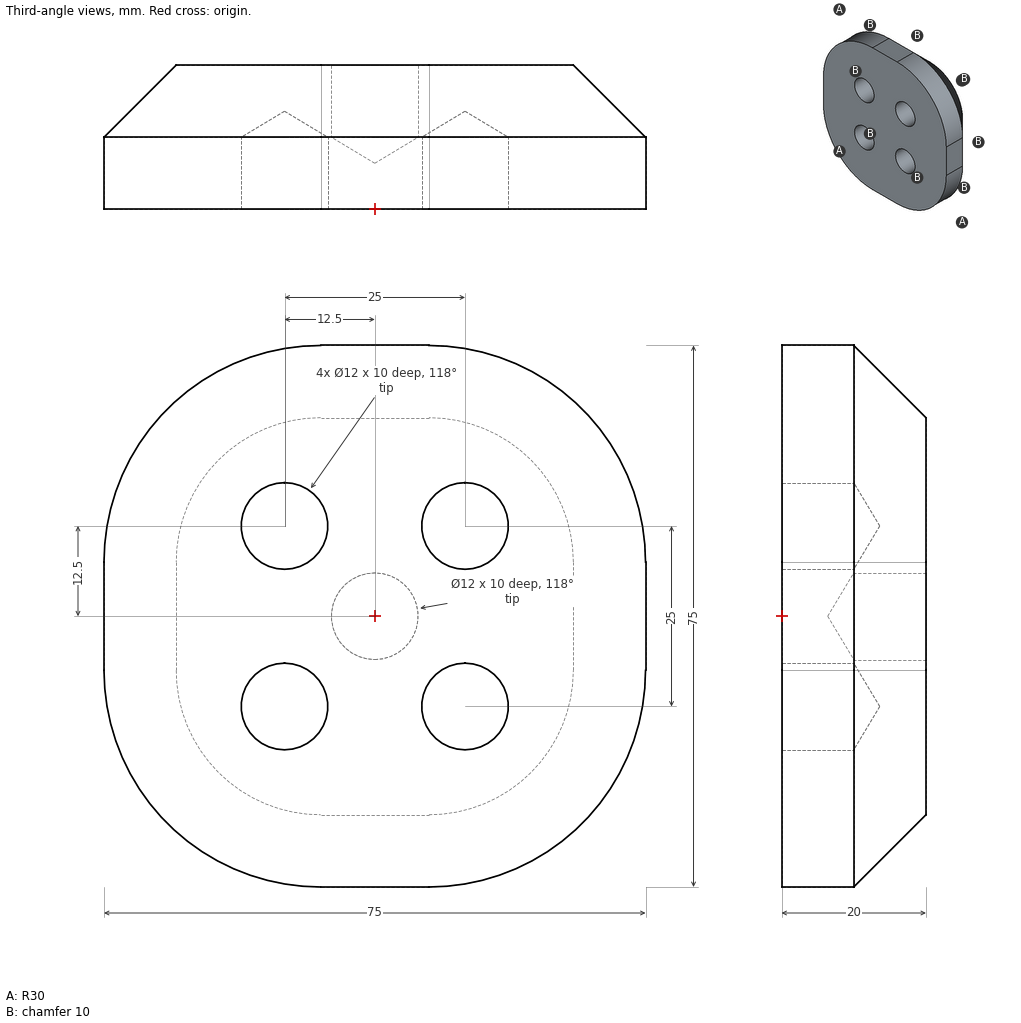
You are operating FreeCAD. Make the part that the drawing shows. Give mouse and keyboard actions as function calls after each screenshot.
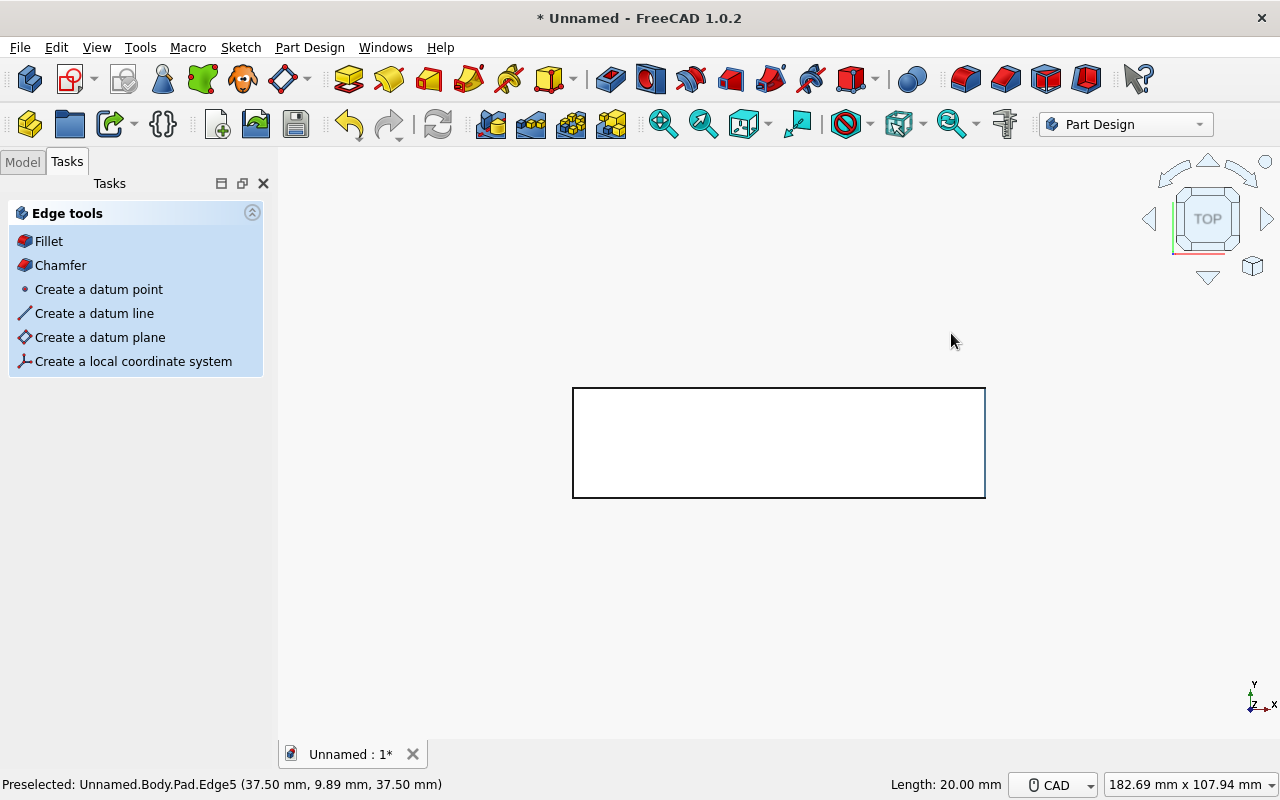
key(v)
key(f)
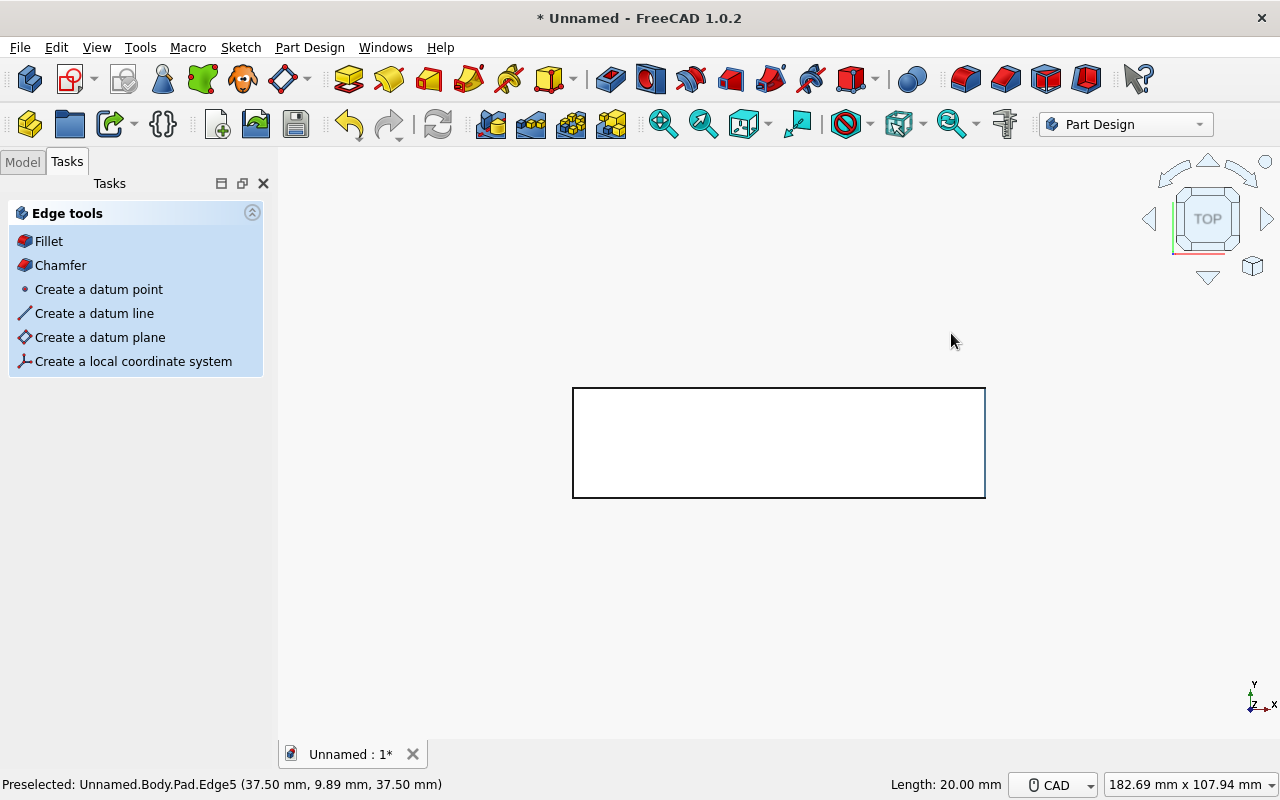
click(573, 442, ctrl)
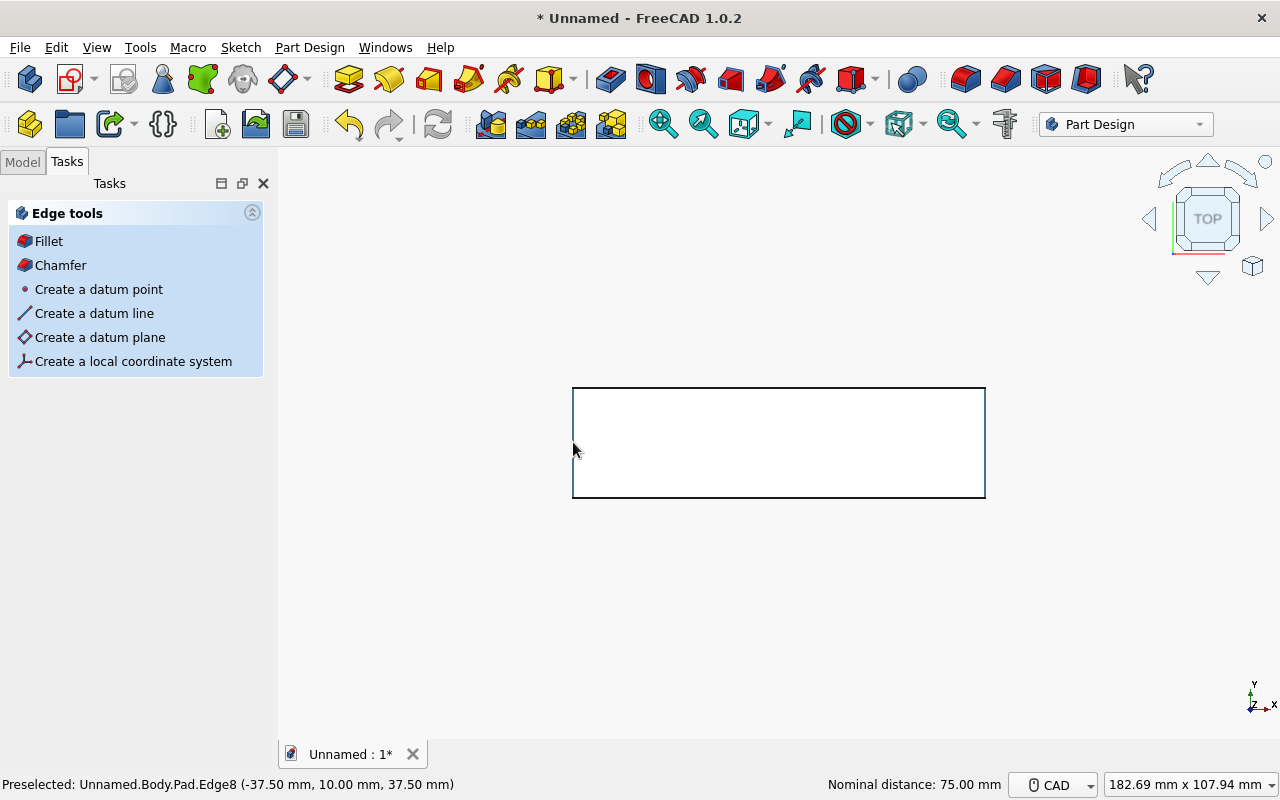
key(1)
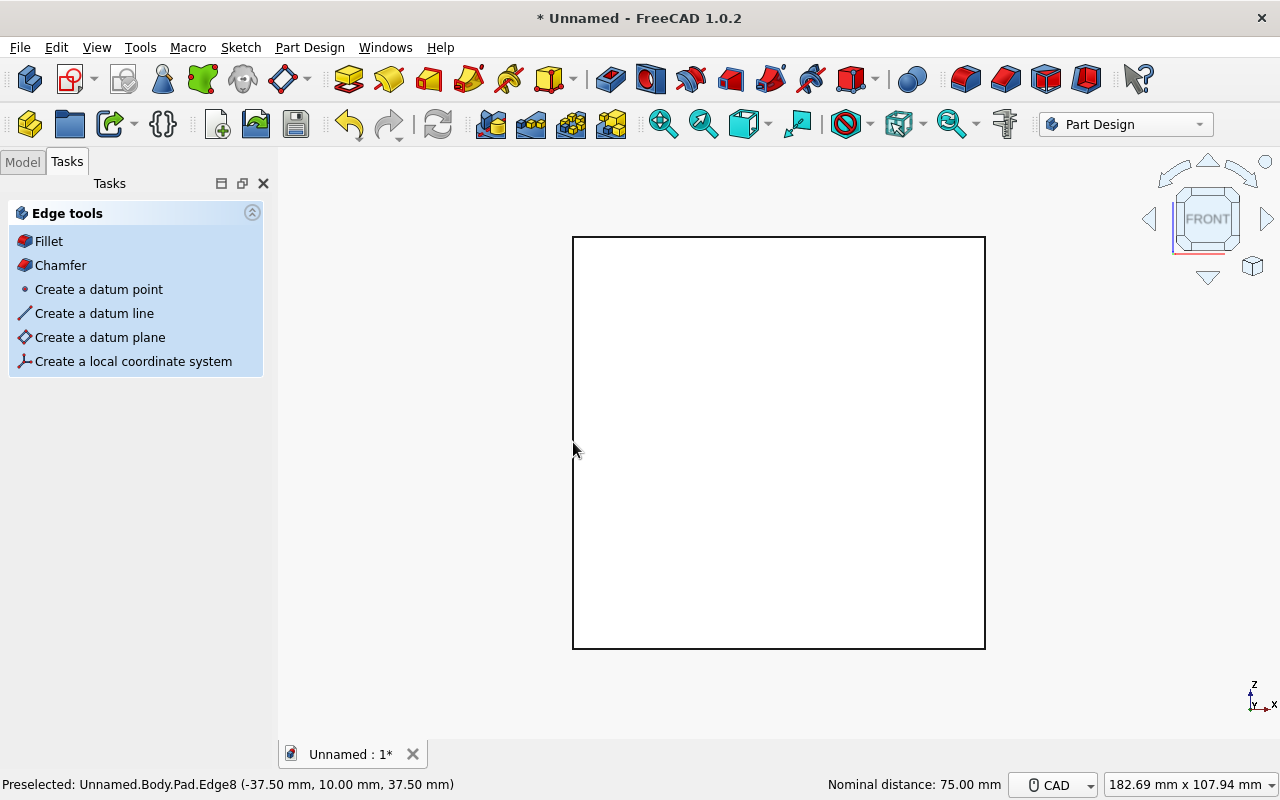
key(3)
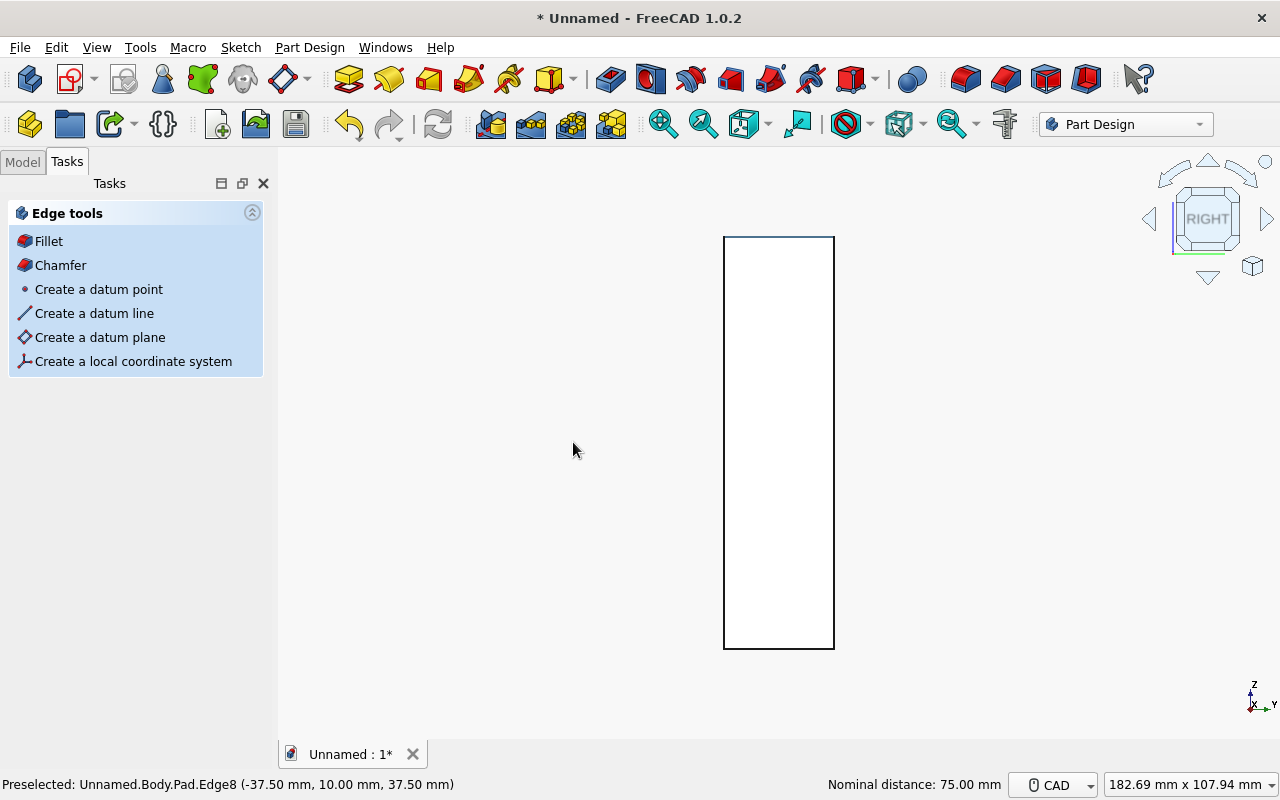
click(779, 648, ctrl)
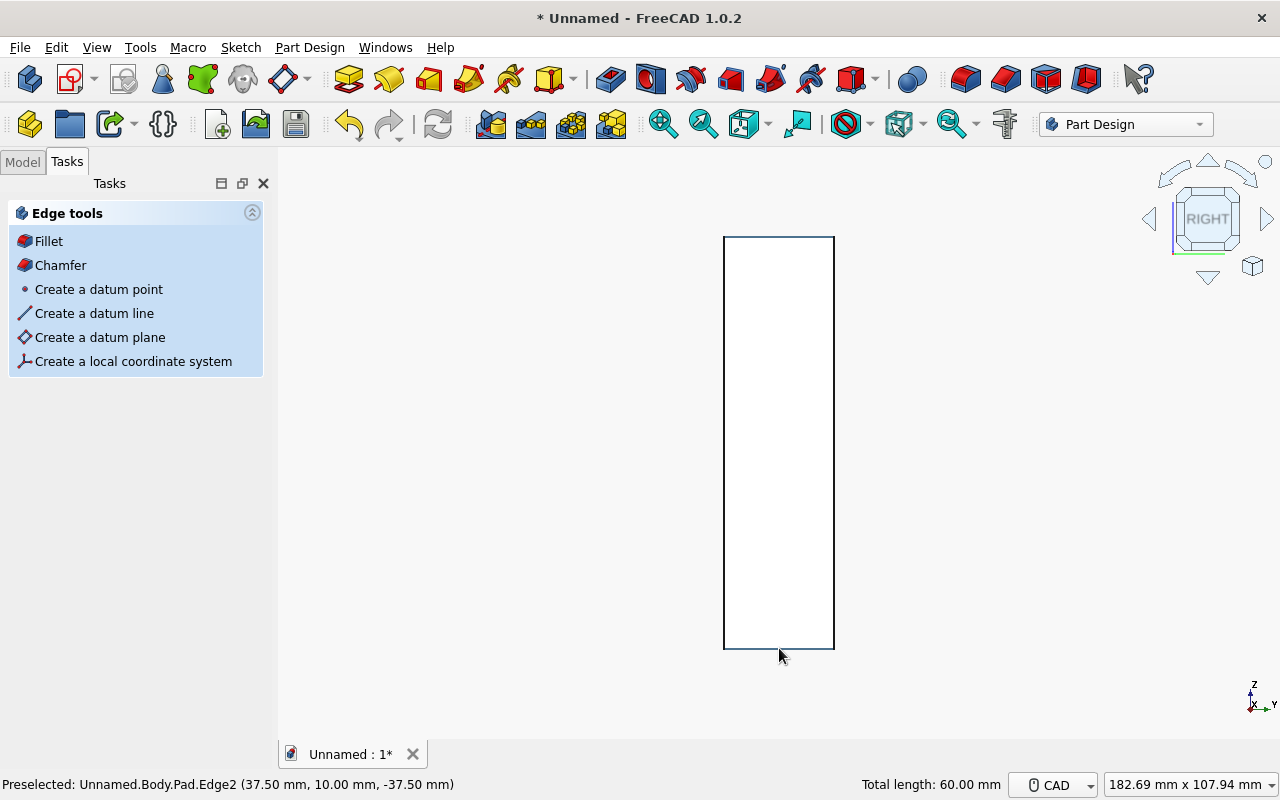
key(5)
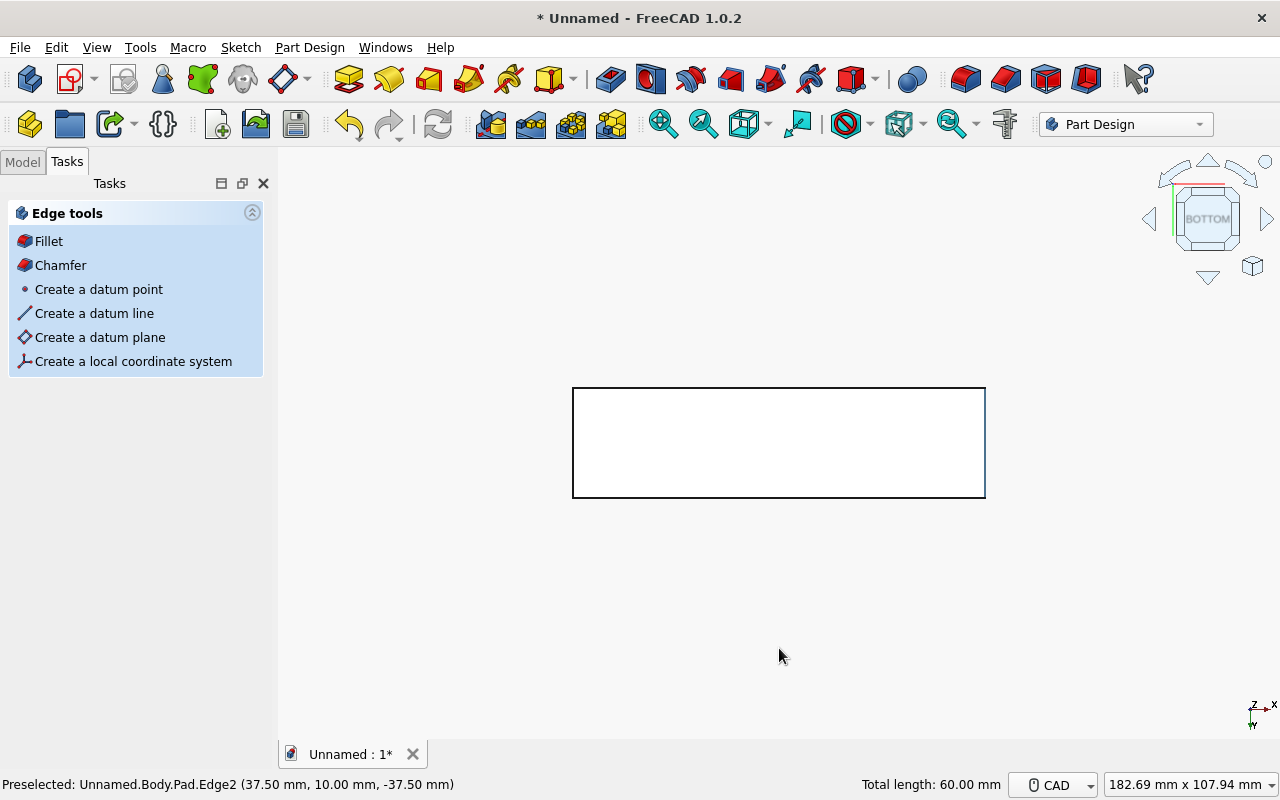
click(664, 124)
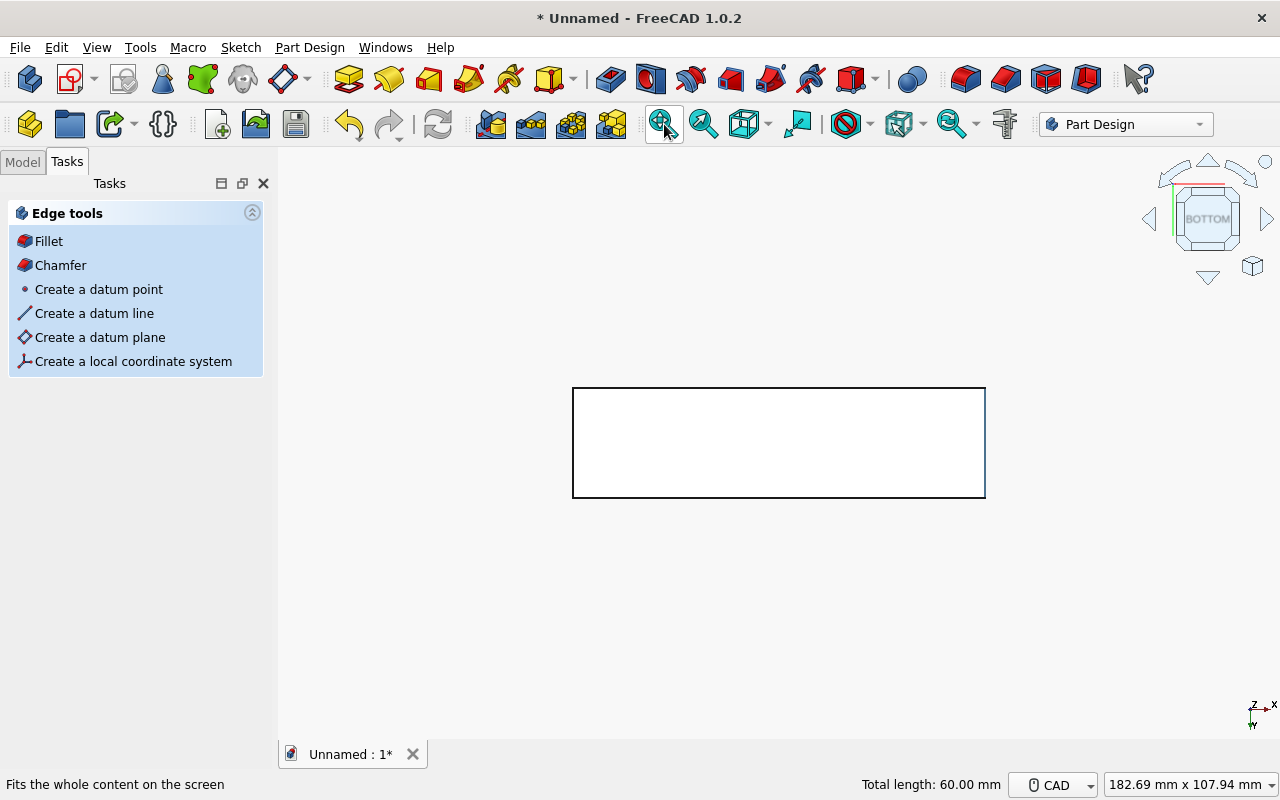
click(573, 442, ctrl)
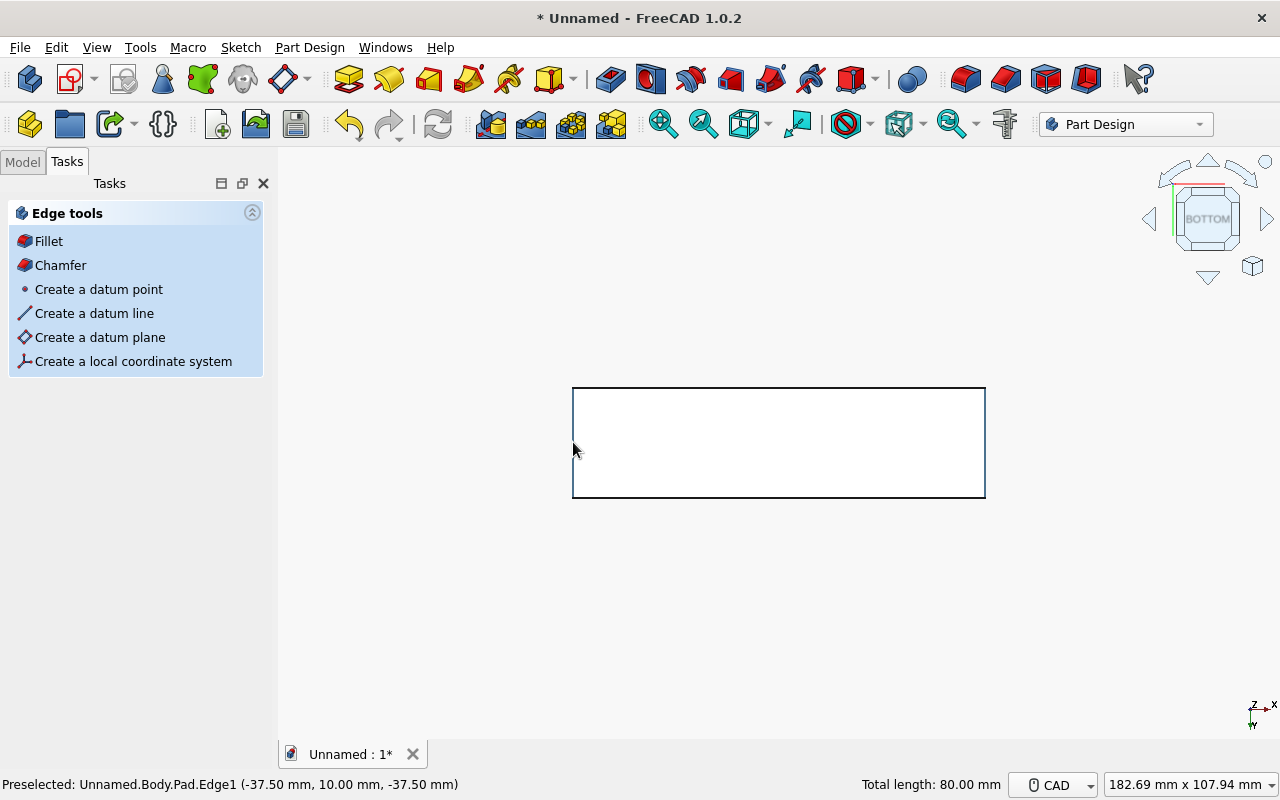
click(966, 80)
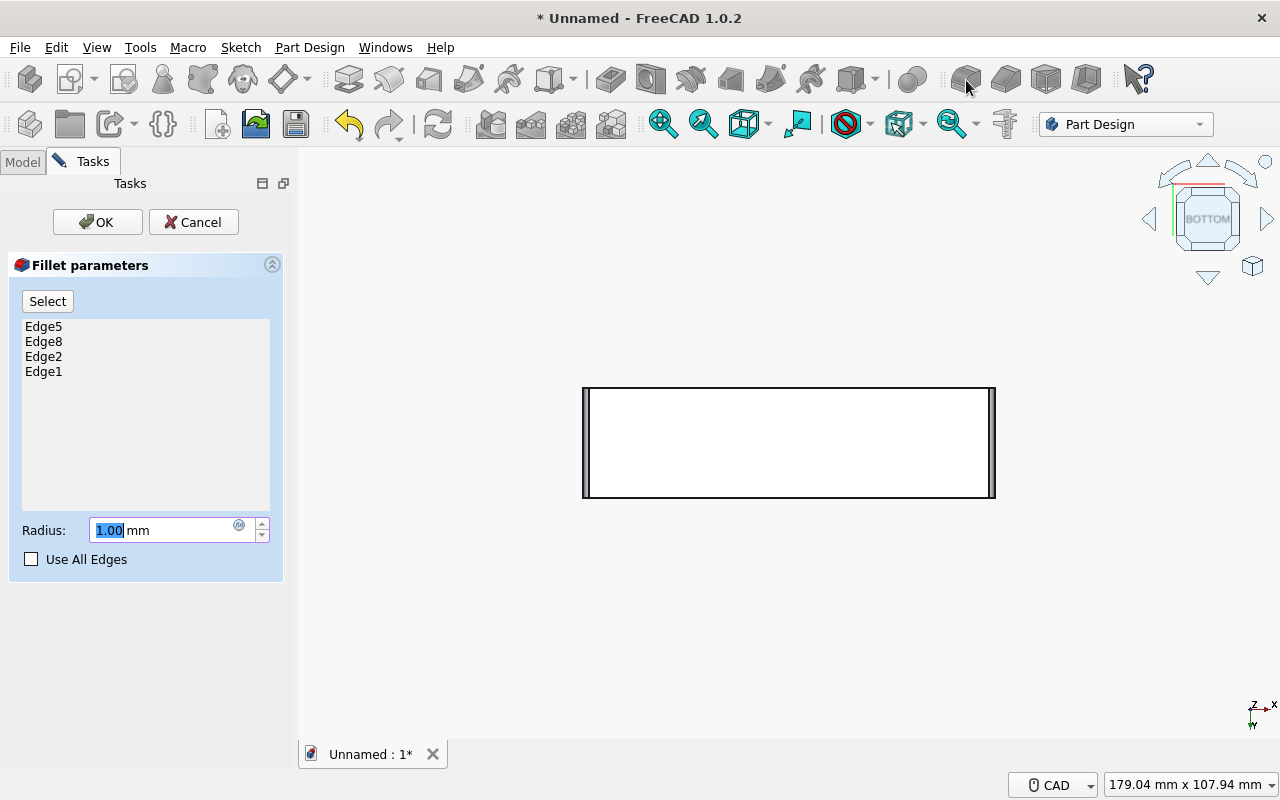
text(30)
key(Tab)